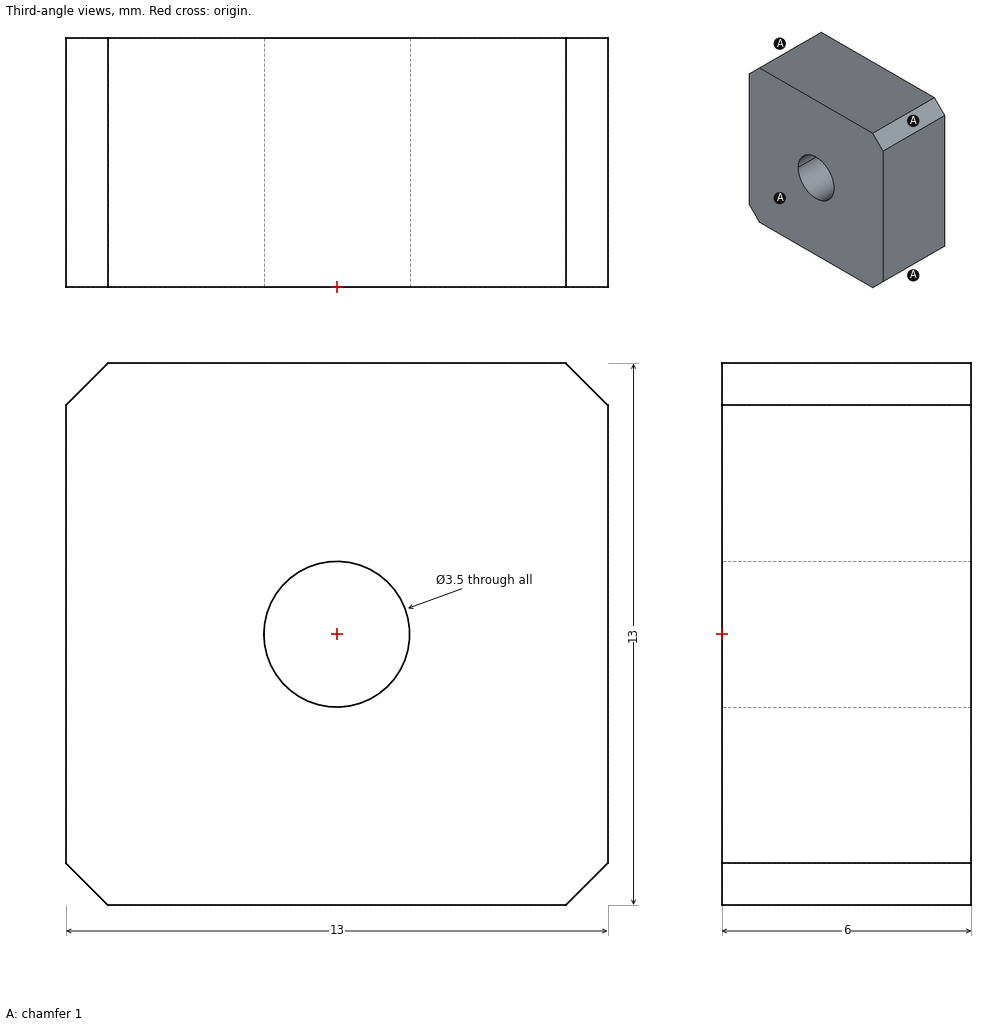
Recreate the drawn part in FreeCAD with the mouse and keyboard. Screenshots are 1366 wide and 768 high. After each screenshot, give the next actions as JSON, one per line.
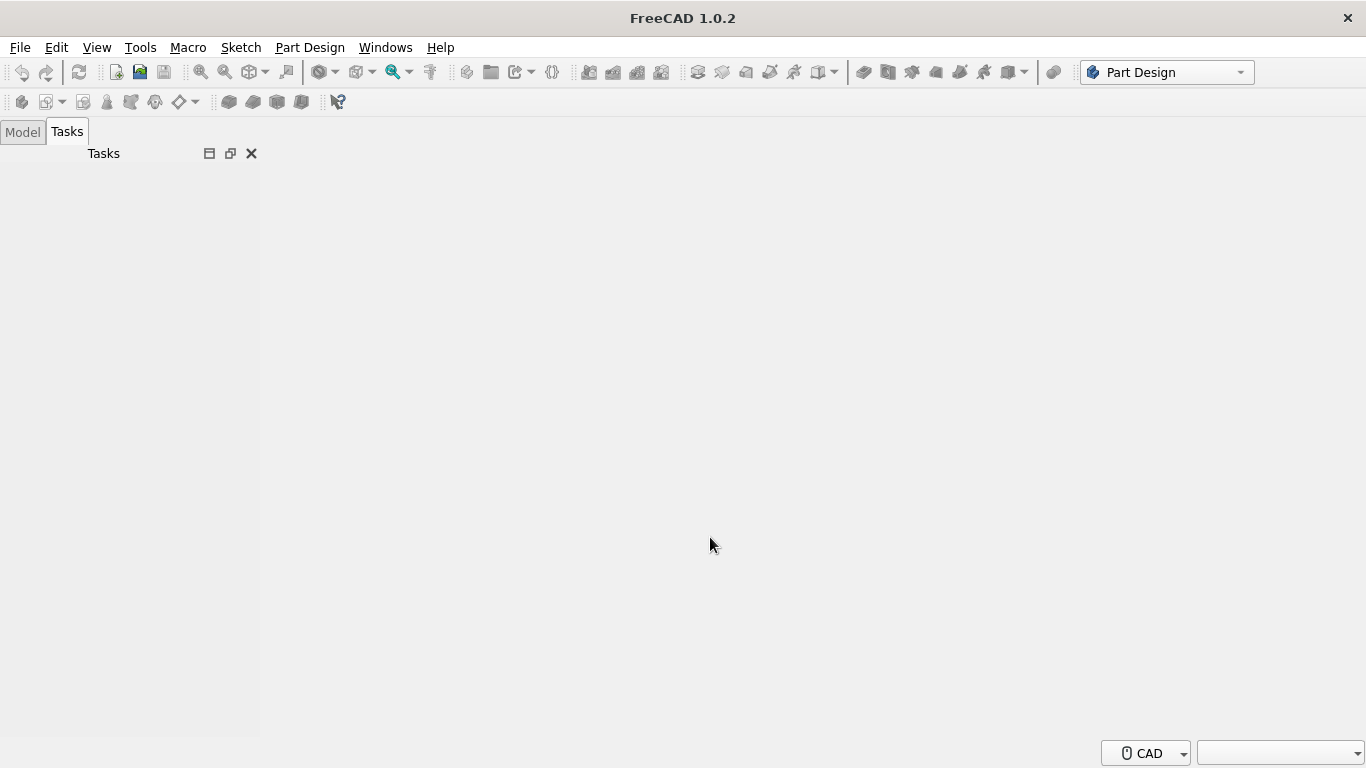
{"action": "key", "text": "ctrl+n"}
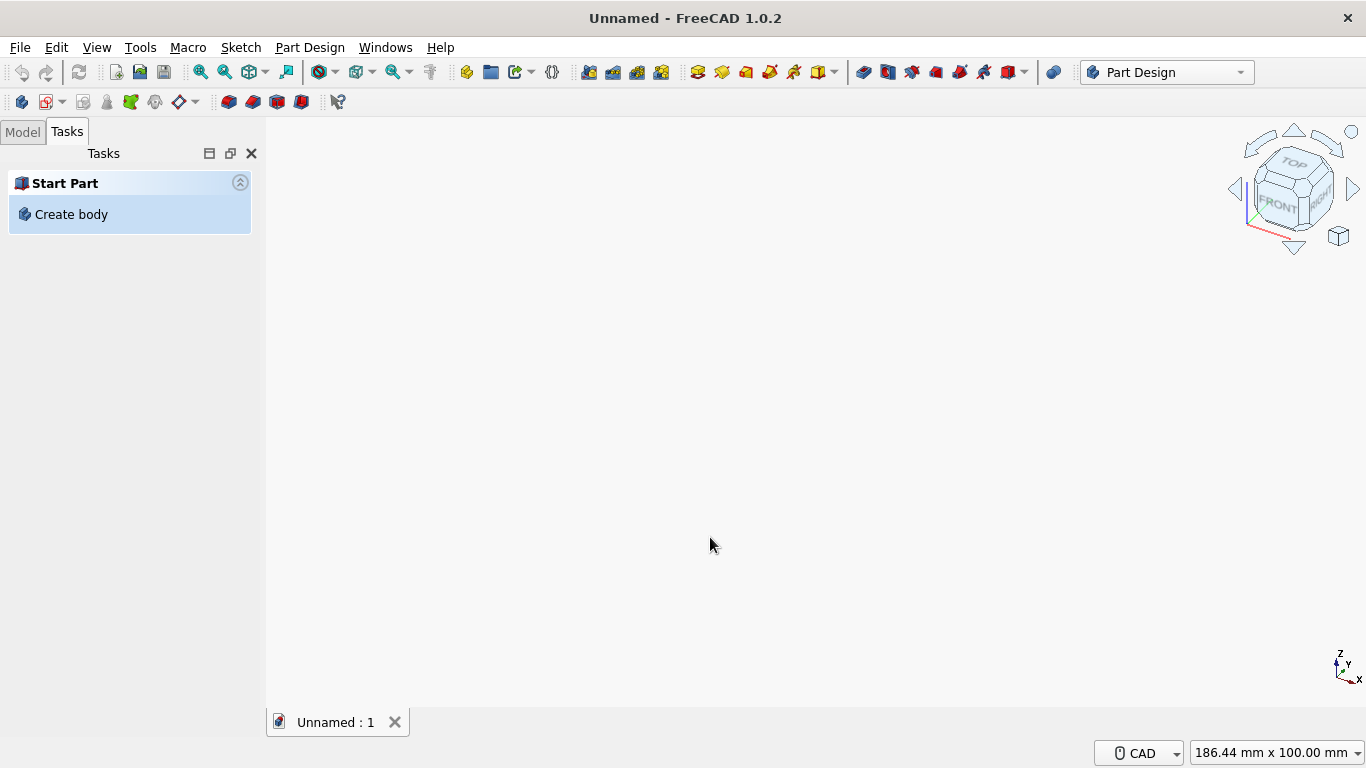
{"action": "left_click", "coordinate": [46, 102]}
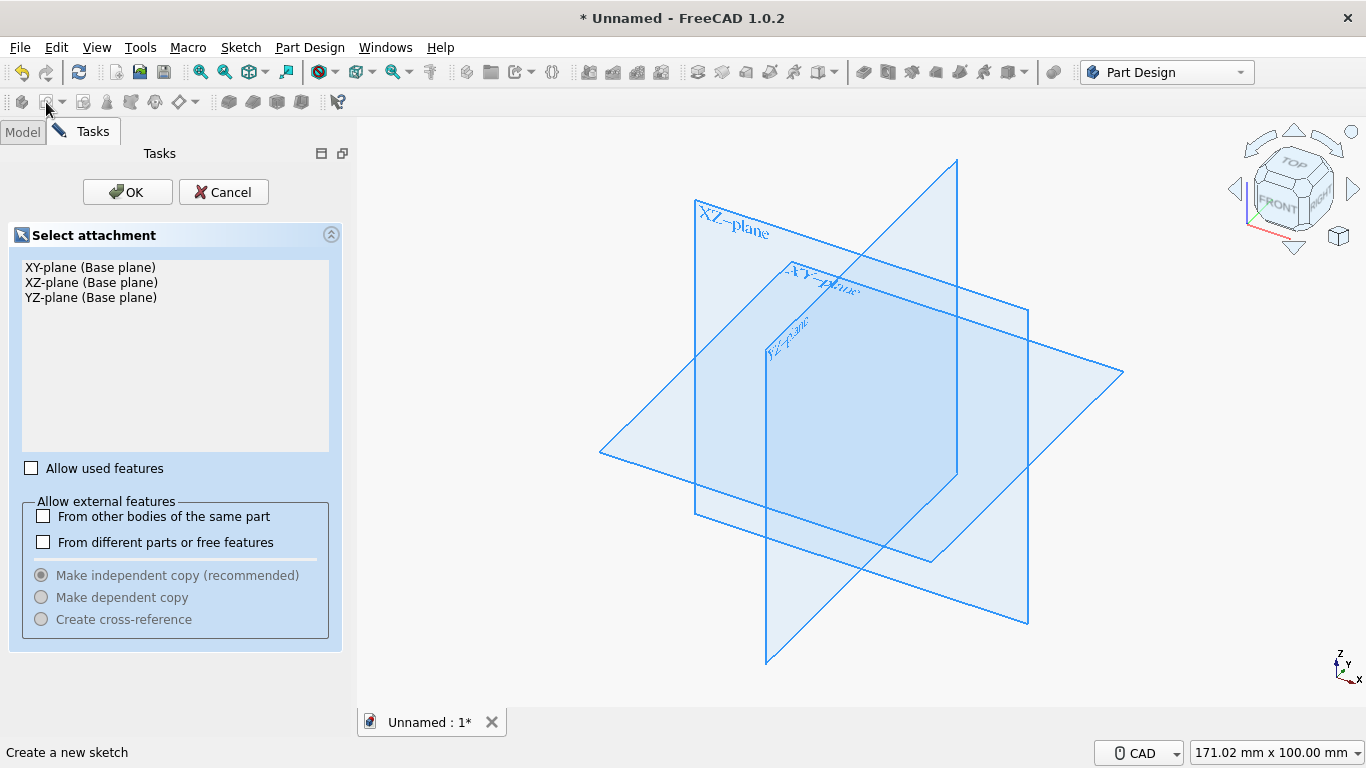
{"action": "left_click", "coordinate": [82, 282]}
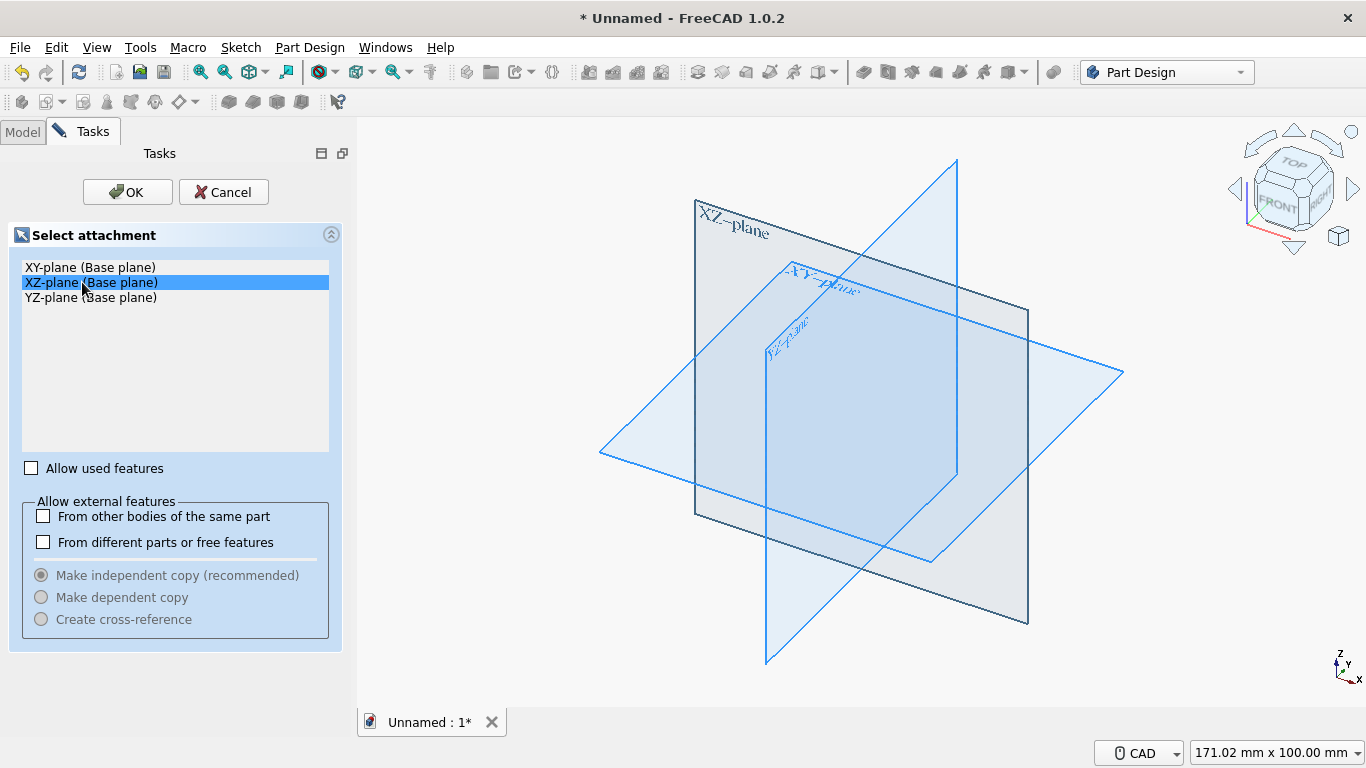
{"action": "left_click", "coordinate": [128, 192]}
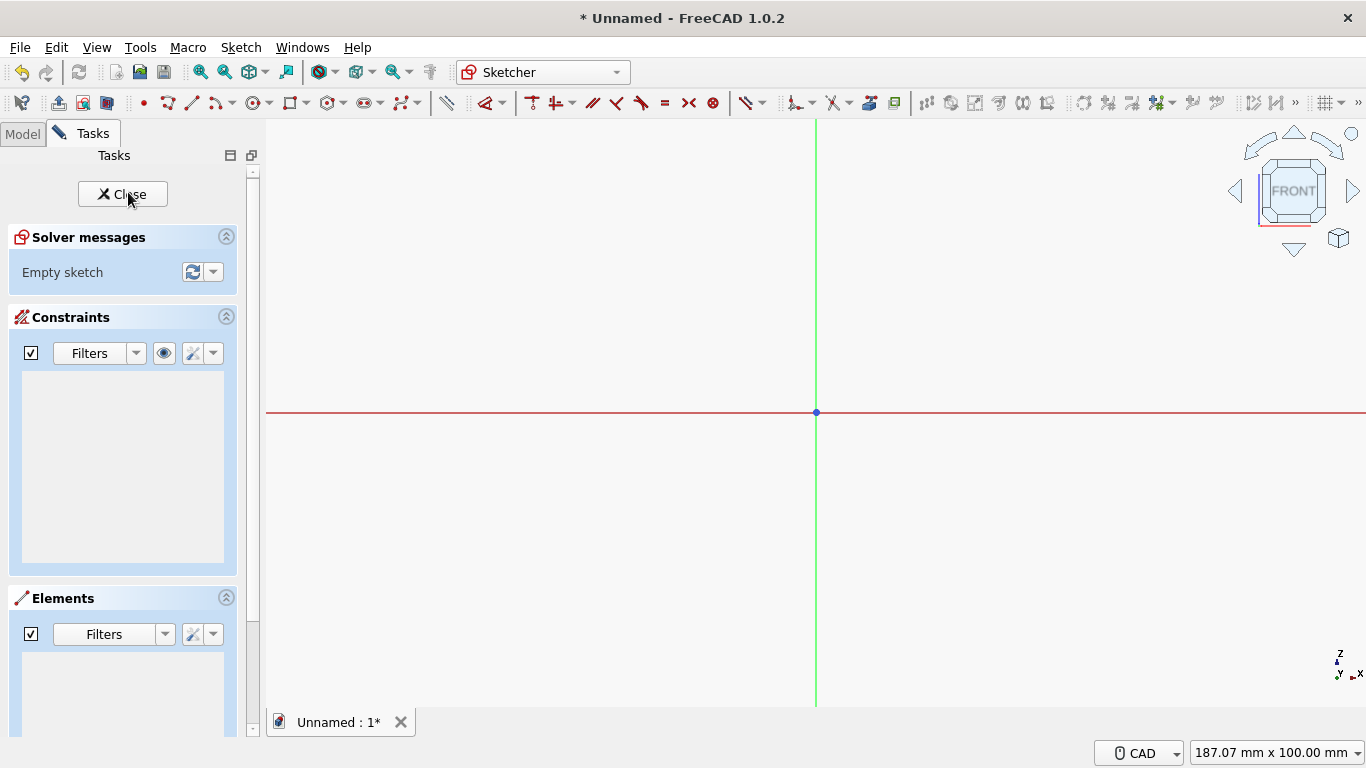
{"action": "scroll", "coordinate": [833, 413], "scroll_direction": "up", "scroll_amount": 8}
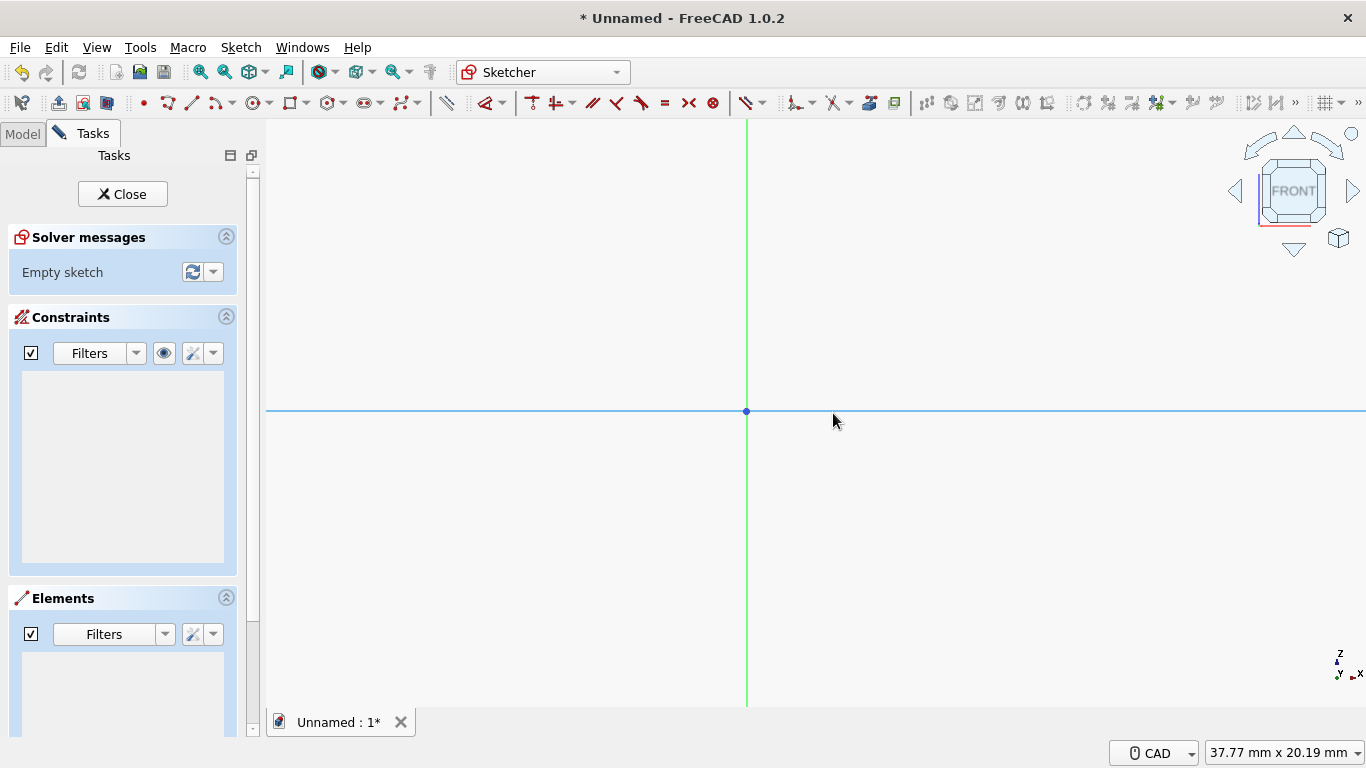
{"action": "key", "text": "g v"}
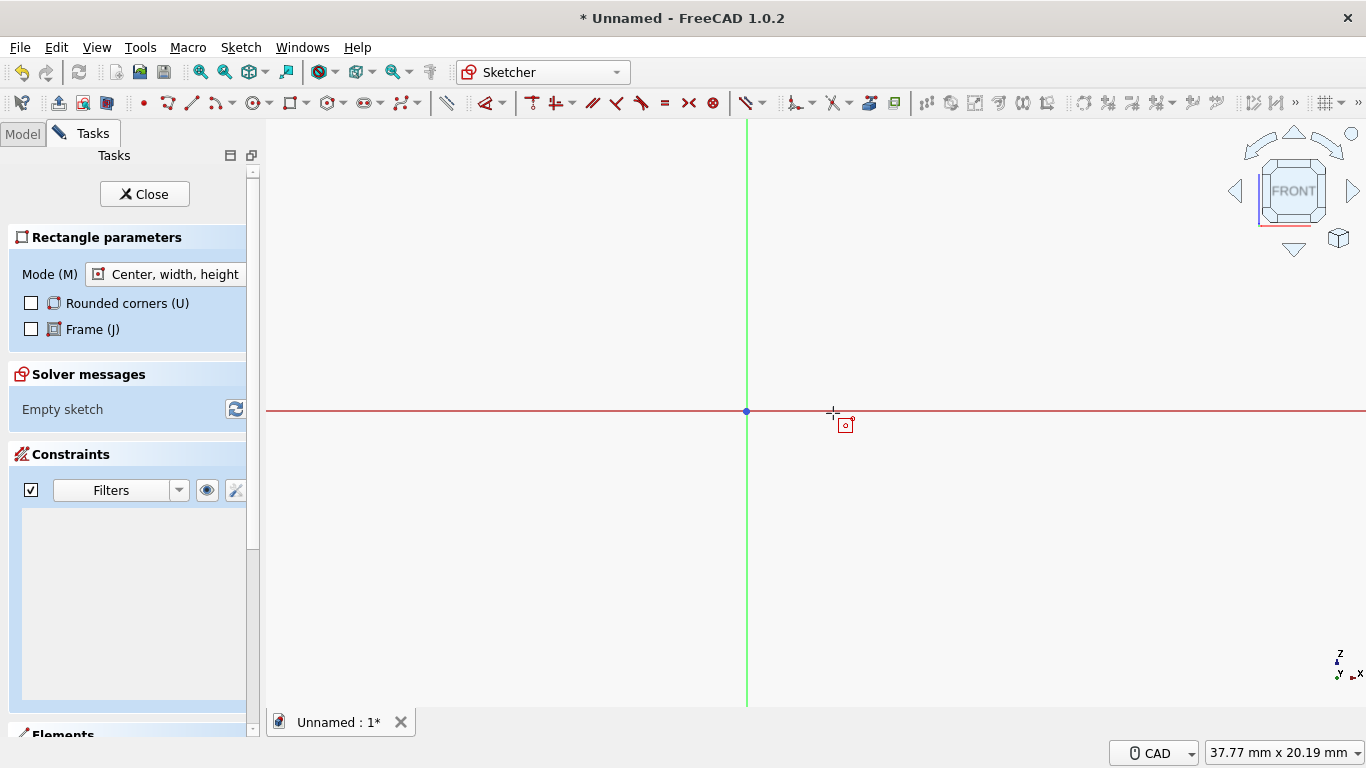
{"action": "left_click", "coordinate": [747, 411]}
{"action": "left_click", "coordinate": [936, 222]}
{"action": "key", "text": "Escape"}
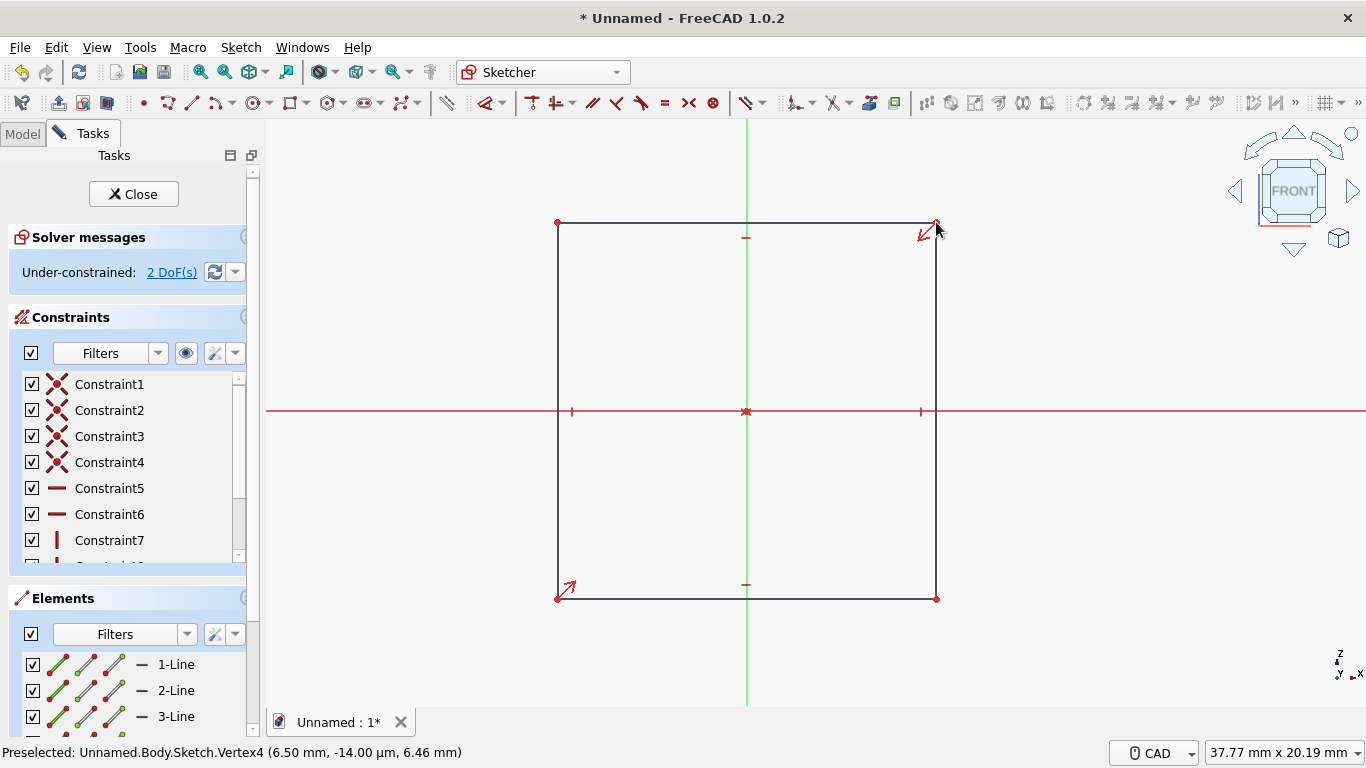
{"action": "key", "text": "d"}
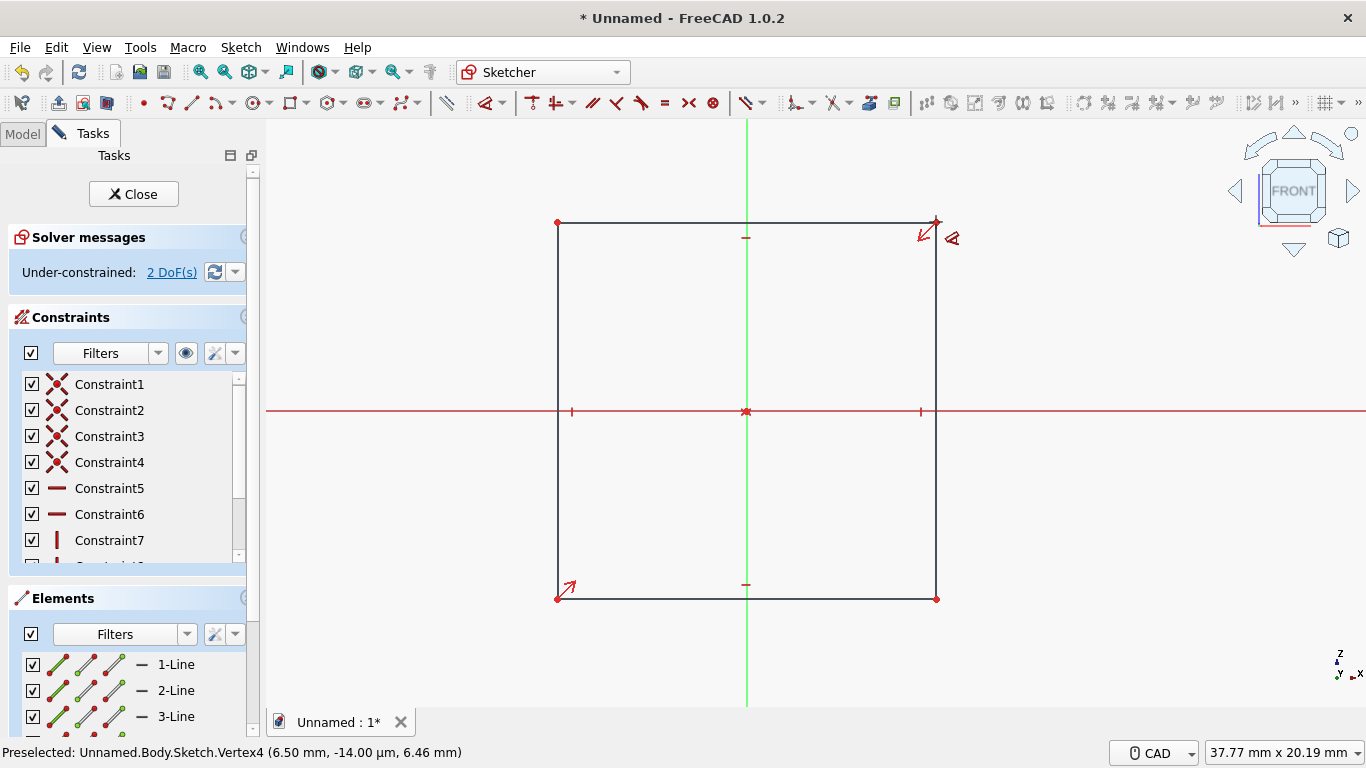
{"action": "left_click", "coordinate": [671, 599]}
{"action": "left_click", "coordinate": [660, 633]}